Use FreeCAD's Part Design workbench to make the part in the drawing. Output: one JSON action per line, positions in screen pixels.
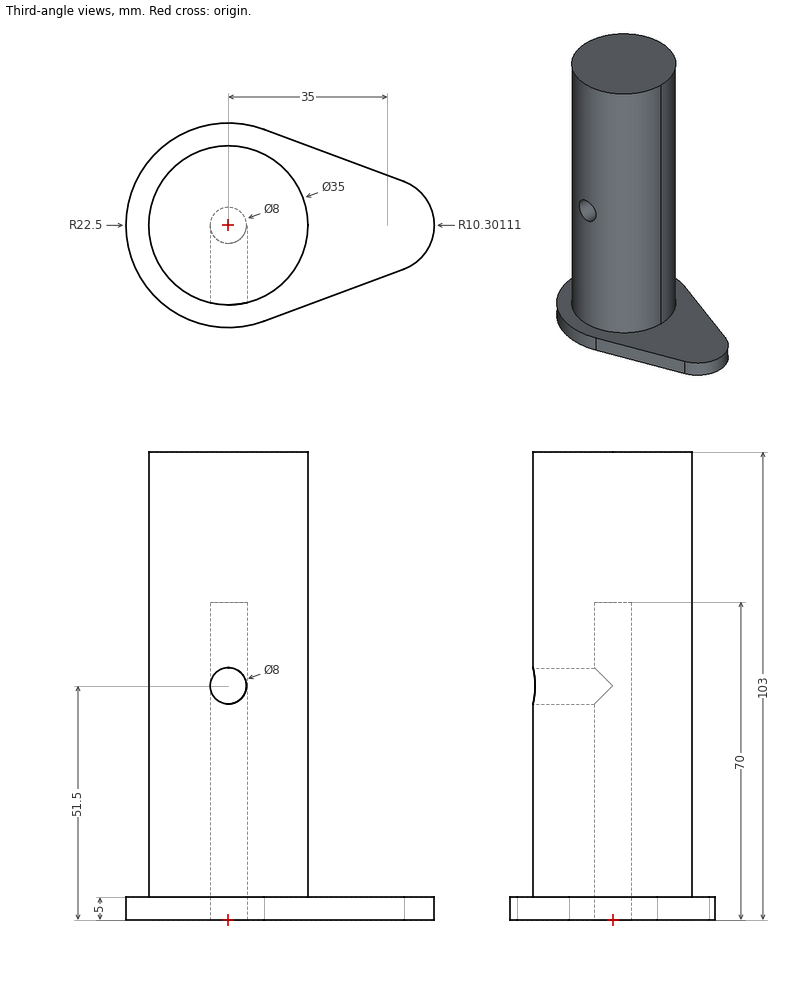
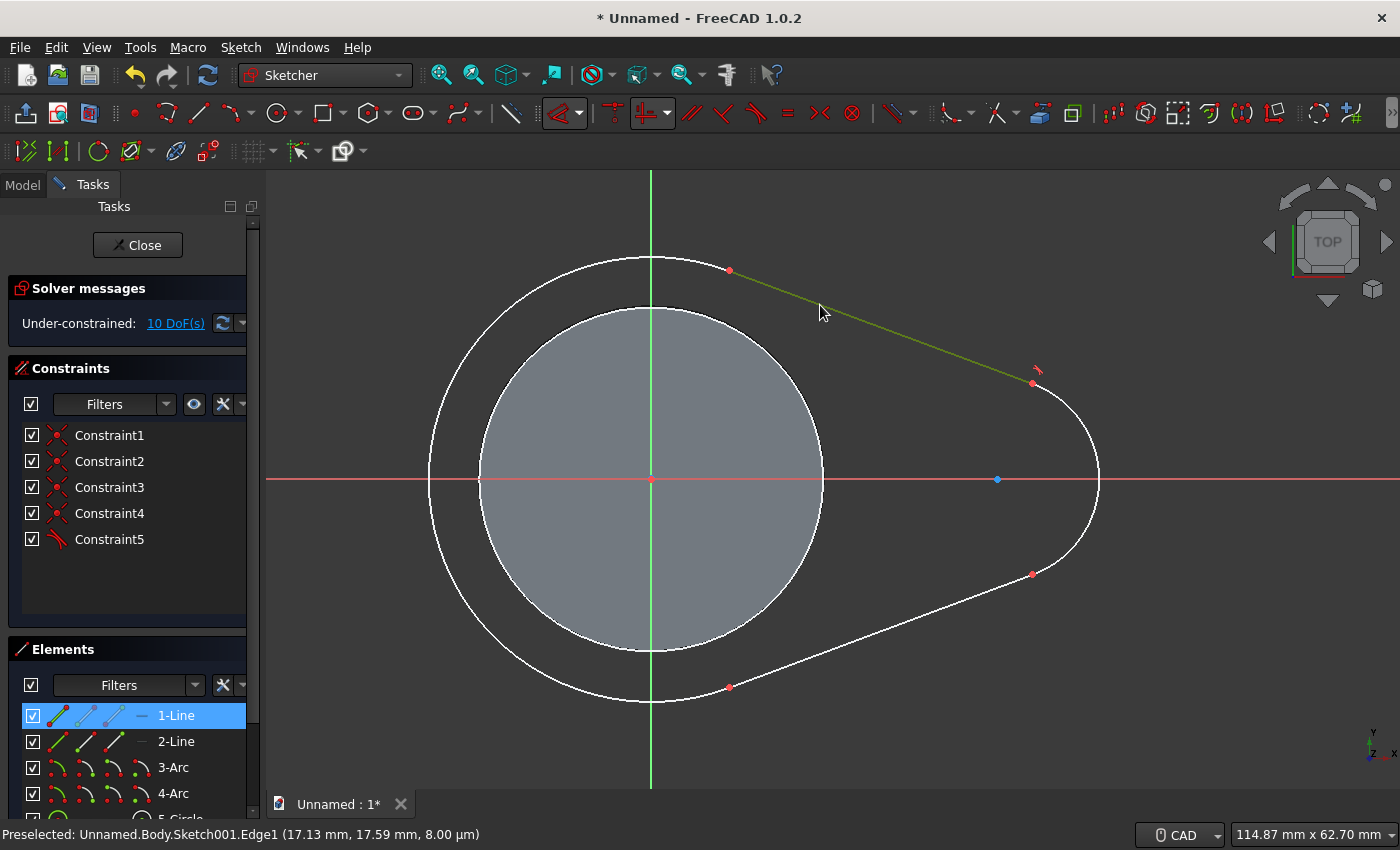
{"action": "left_click", "coordinate": [492, 324]}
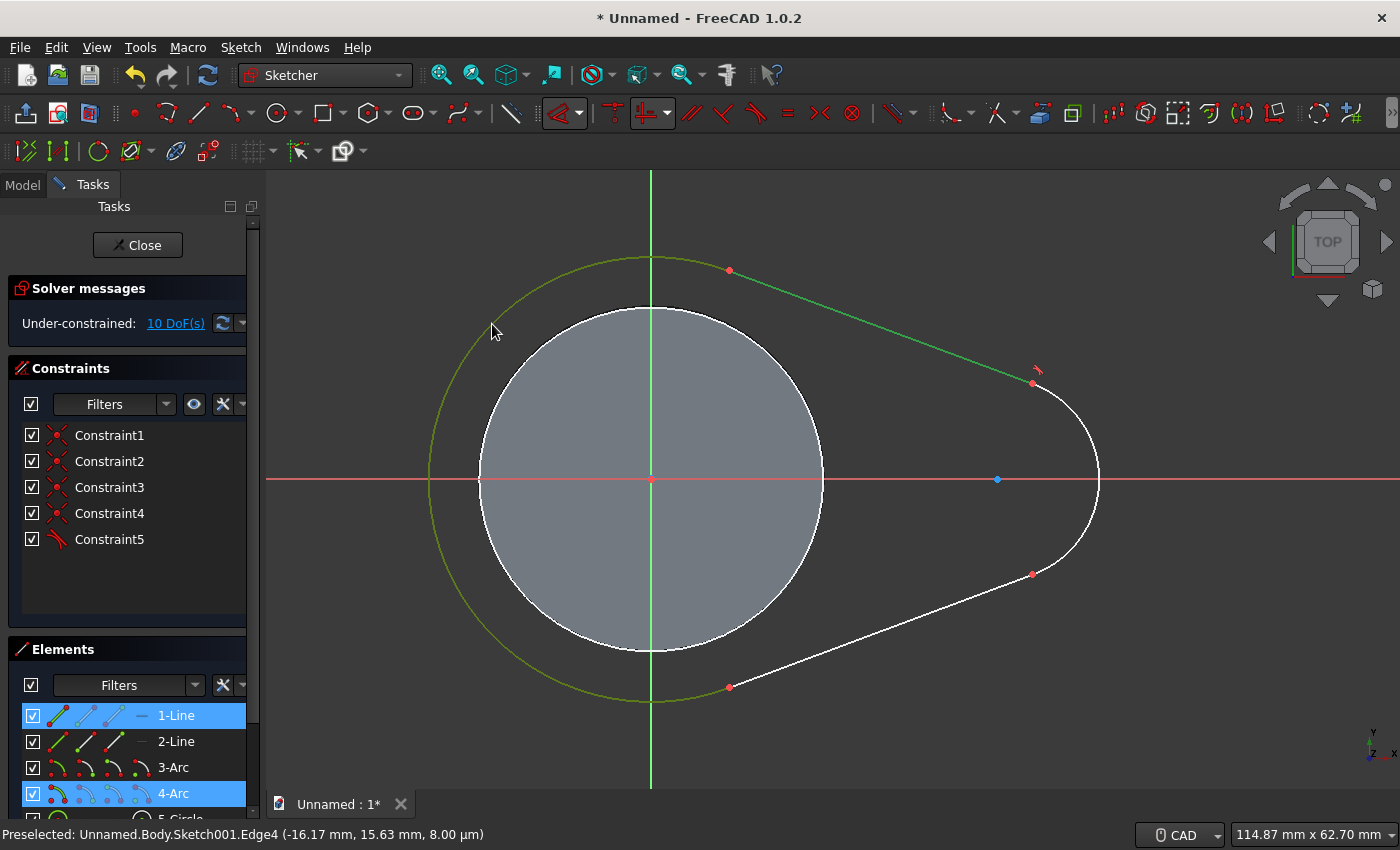
{"action": "left_click", "coordinate": [756, 114]}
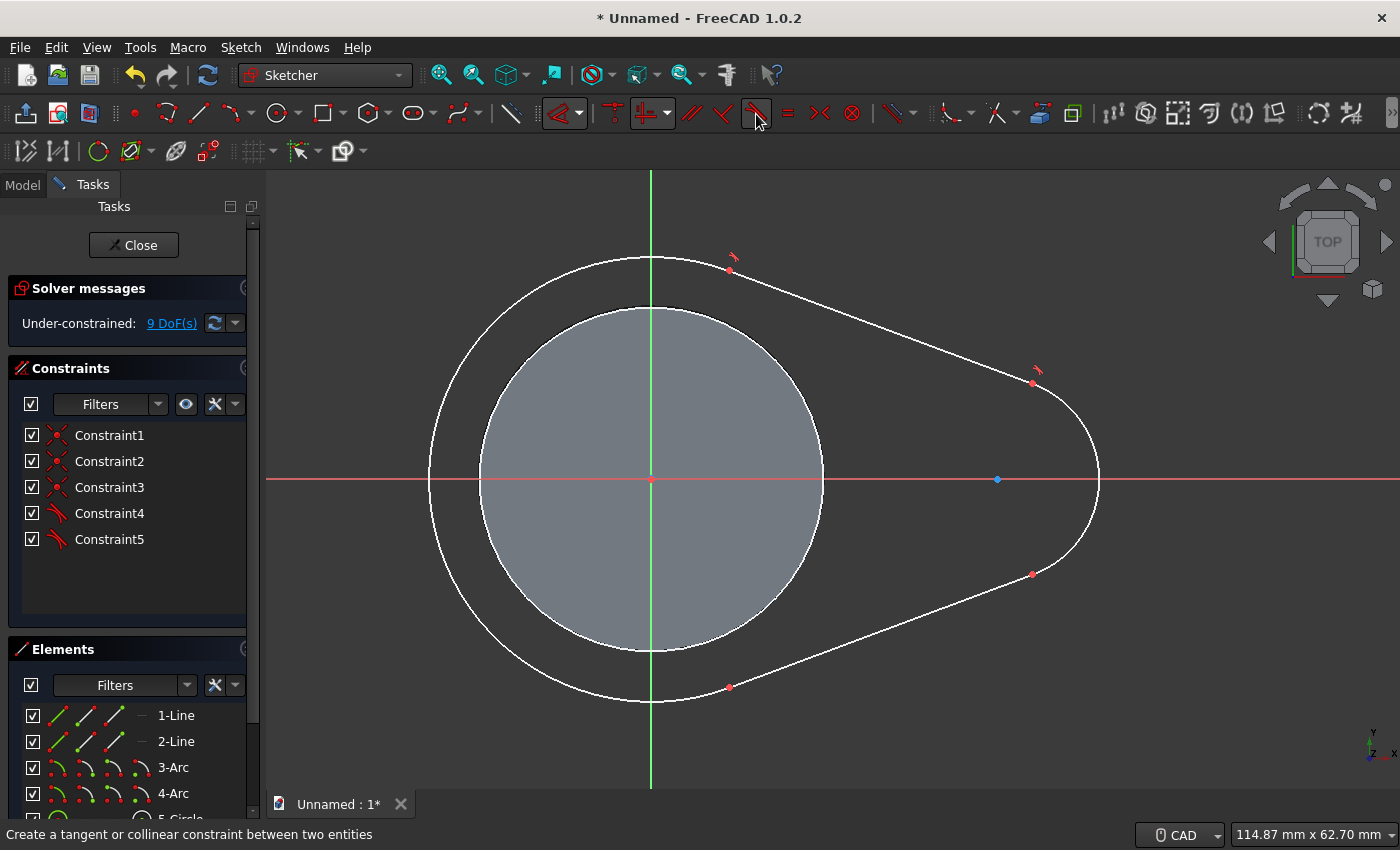
{"action": "left_click", "coordinate": [941, 609]}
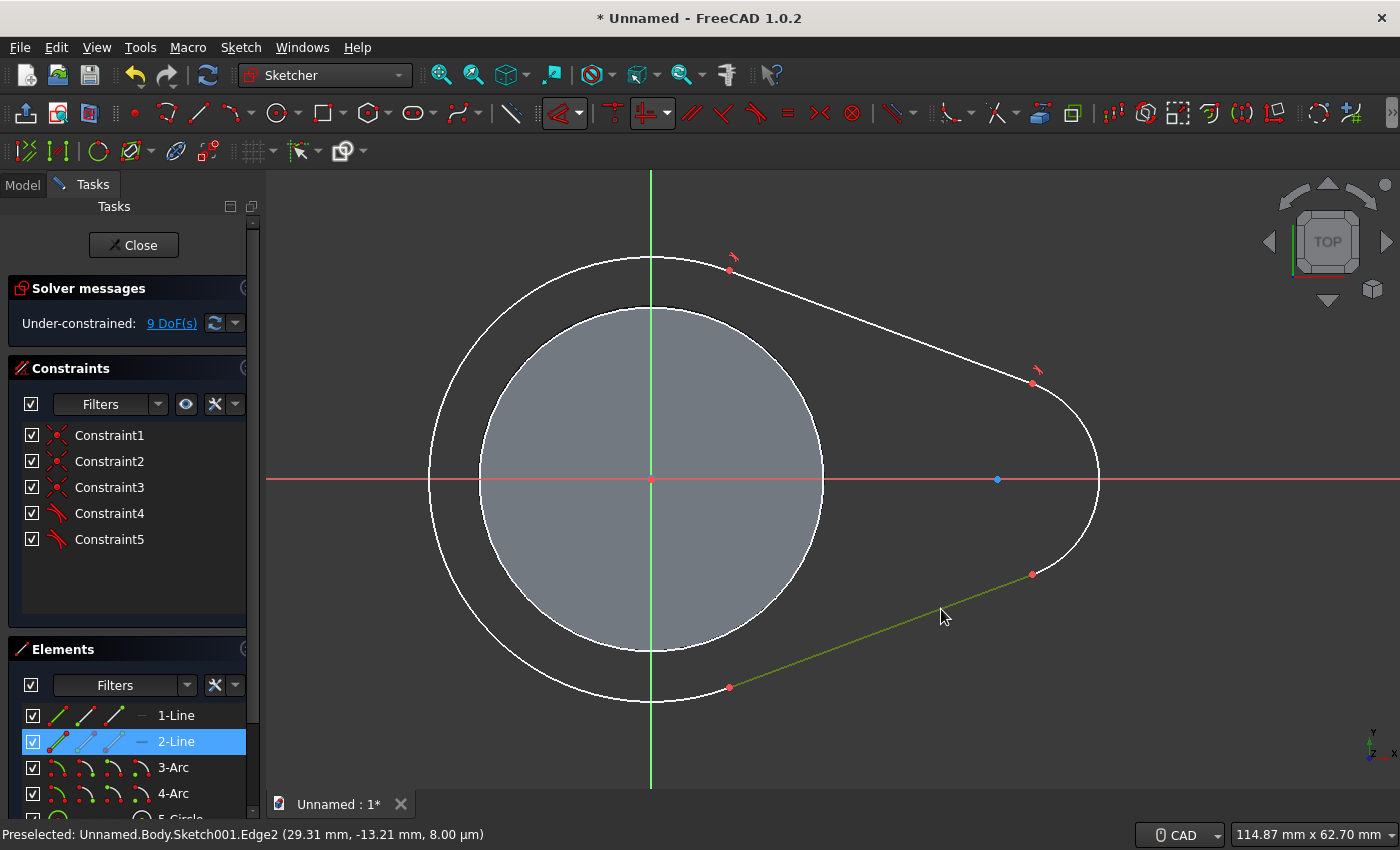
{"action": "left_click", "coordinate": [1087, 527]}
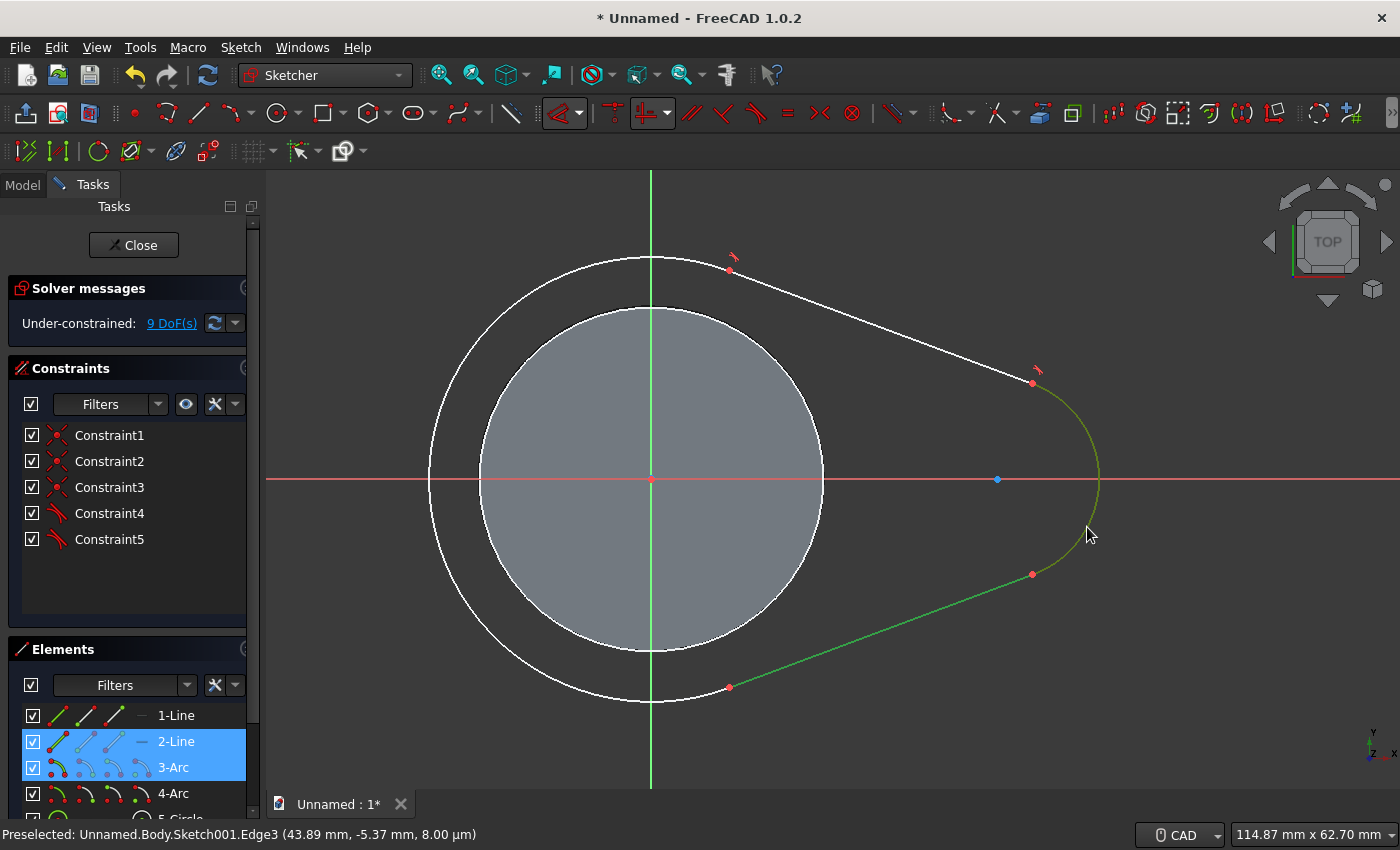
{"action": "left_click", "coordinate": [756, 114]}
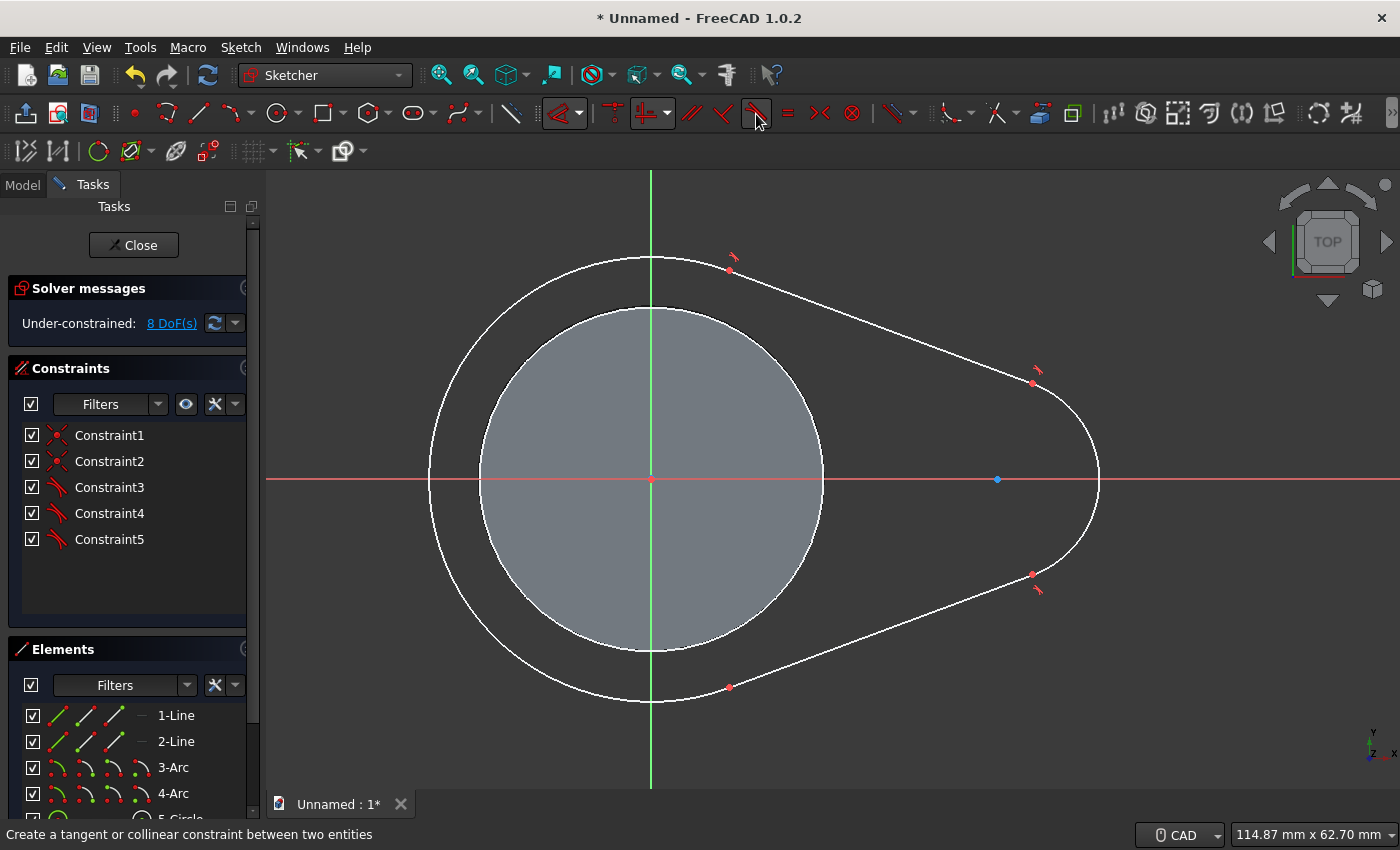
{"action": "left_click", "coordinate": [942, 609]}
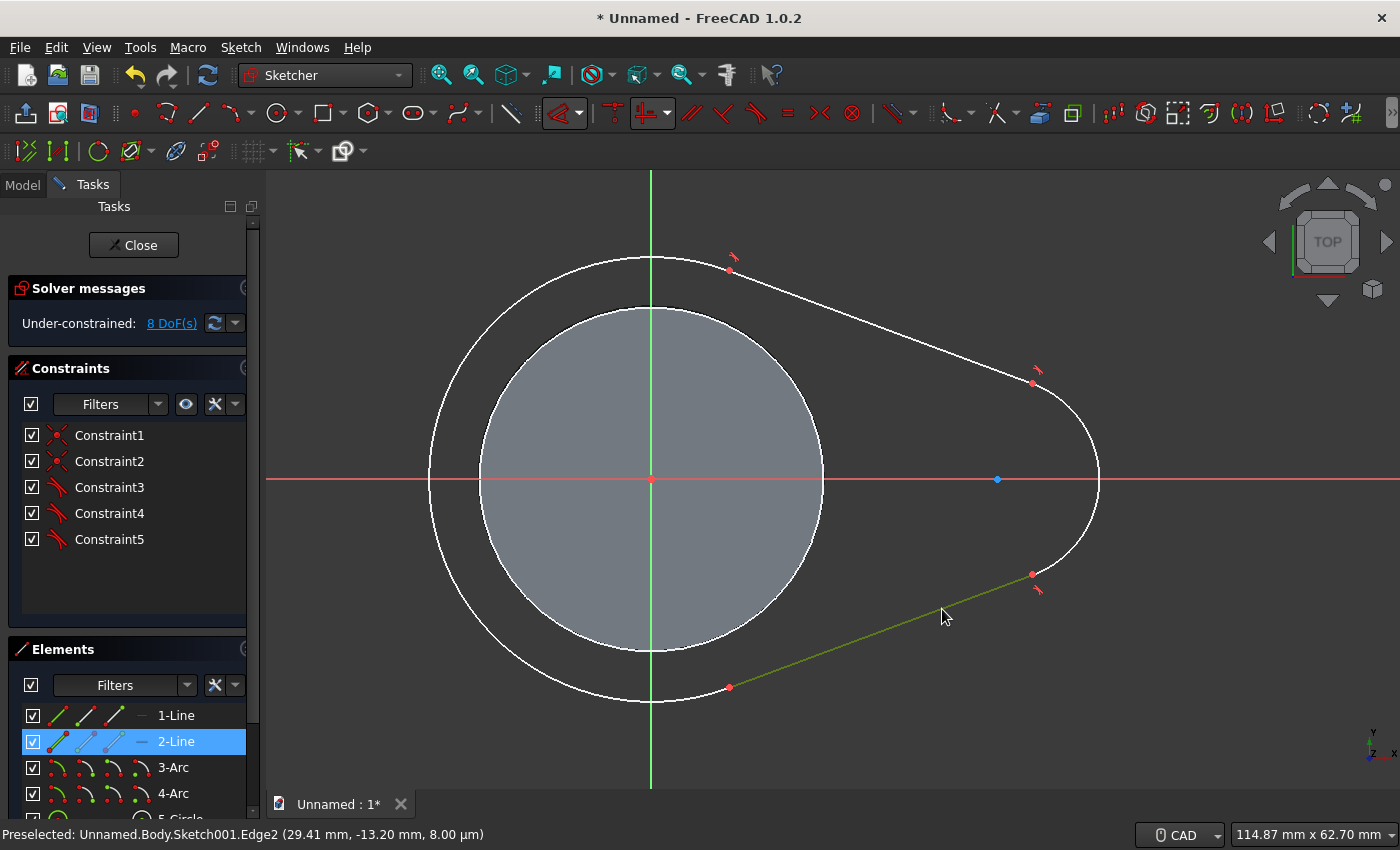
{"action": "left_click", "coordinate": [492, 325]}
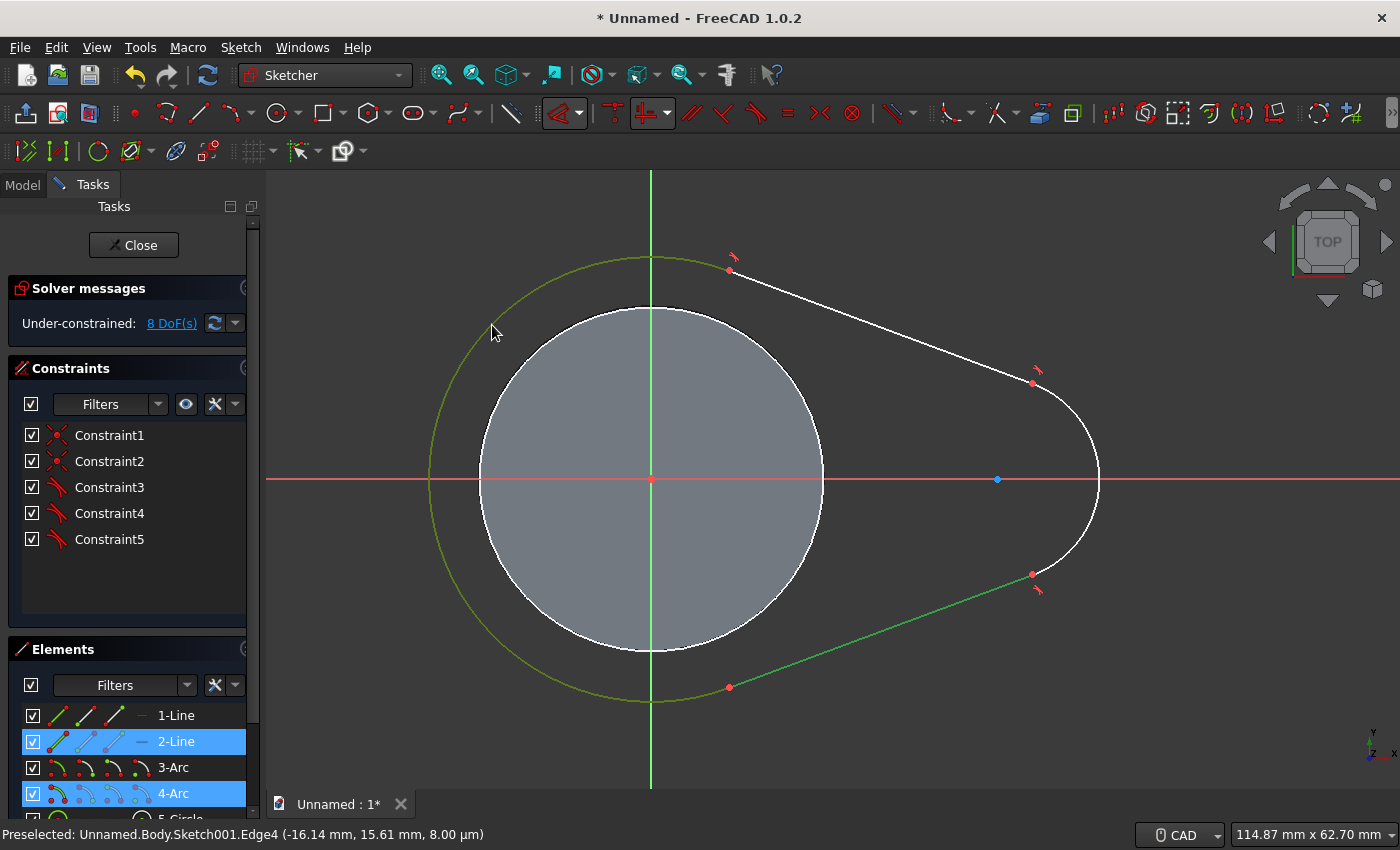
{"action": "left_click", "coordinate": [756, 114]}